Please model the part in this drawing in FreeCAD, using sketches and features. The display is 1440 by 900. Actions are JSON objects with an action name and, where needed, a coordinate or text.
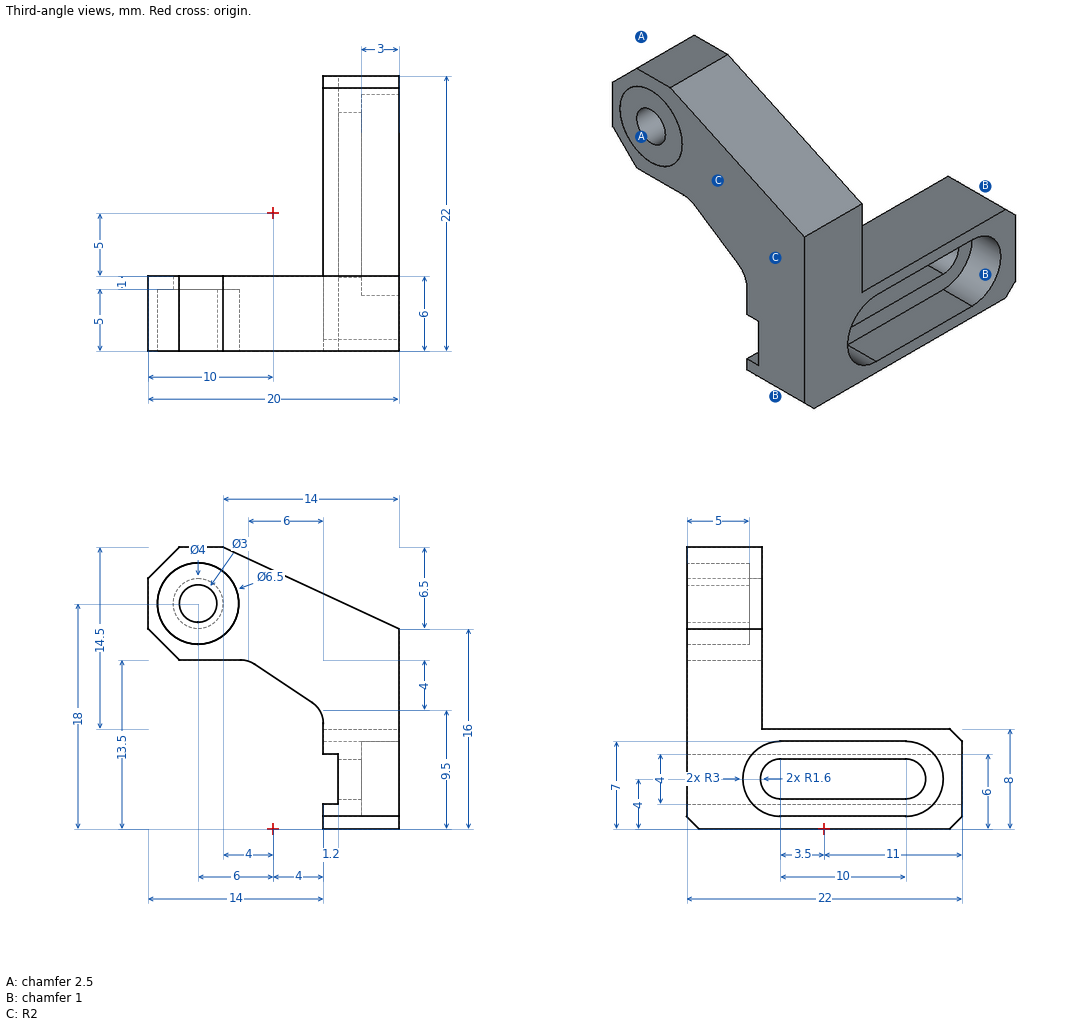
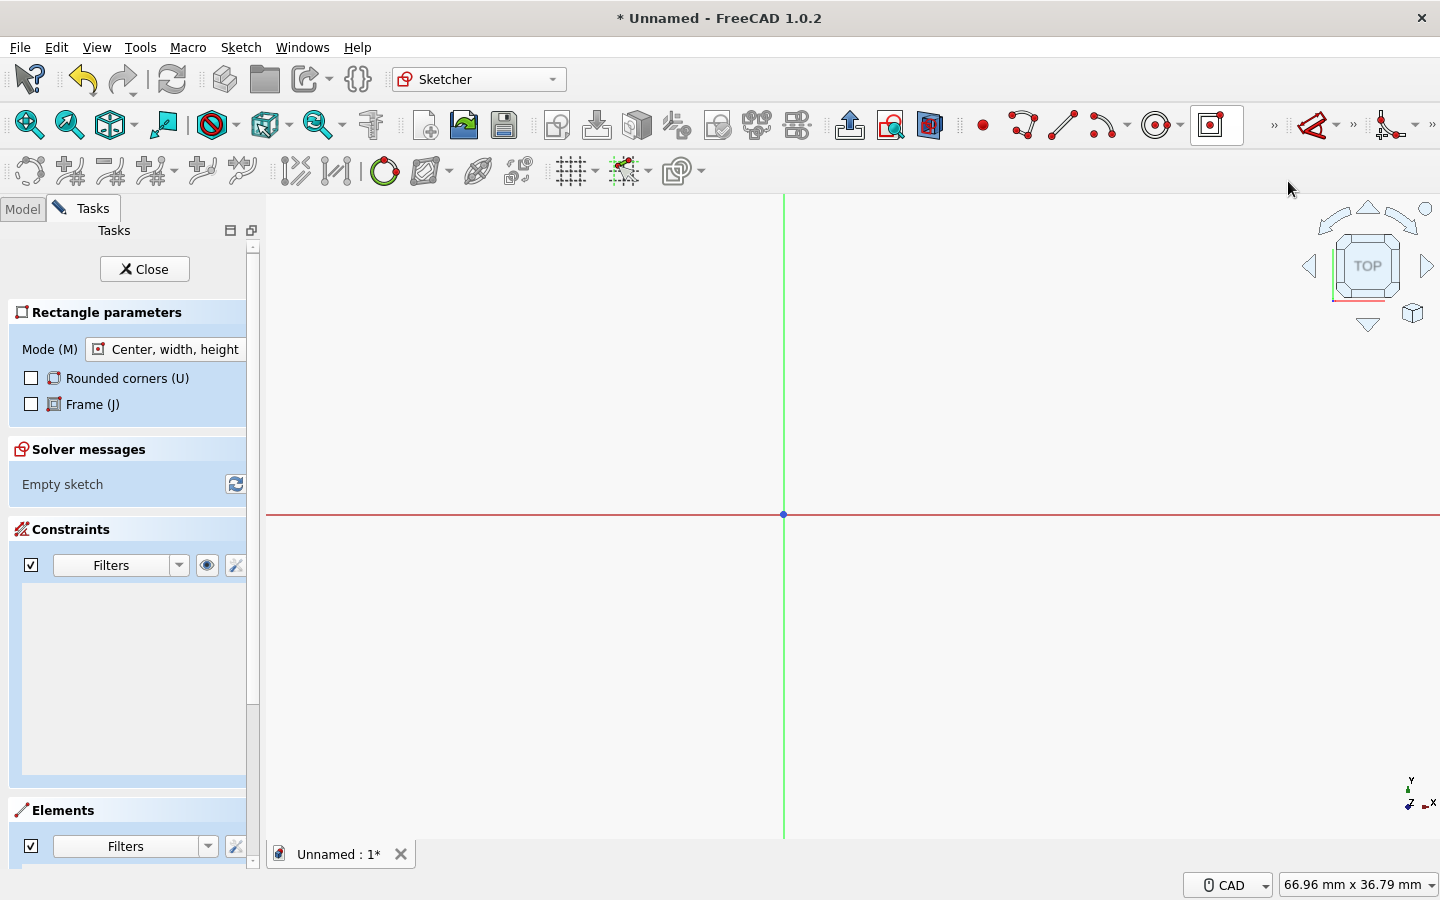
{"action": "left_click", "coordinate": [784, 515]}
{"action": "mouse_move", "coordinate": [959, 322]}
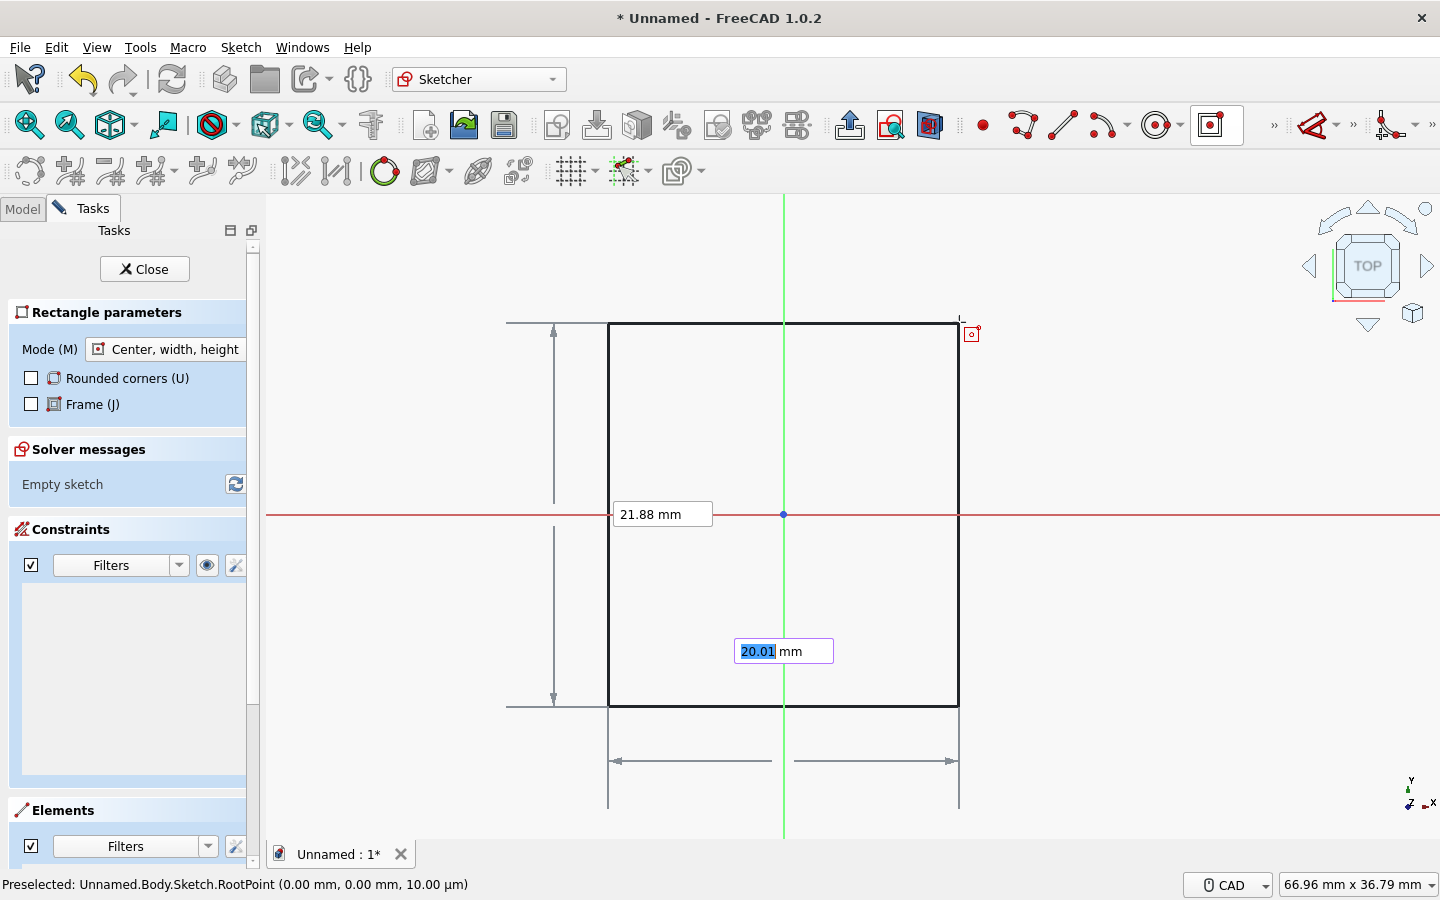
{"action": "type", "text": "20"}
{"action": "key", "text": "Tab"}
{"action": "type", "text": "22"}
{"action": "key", "text": "Return"}
{"action": "key", "text": "Escape"}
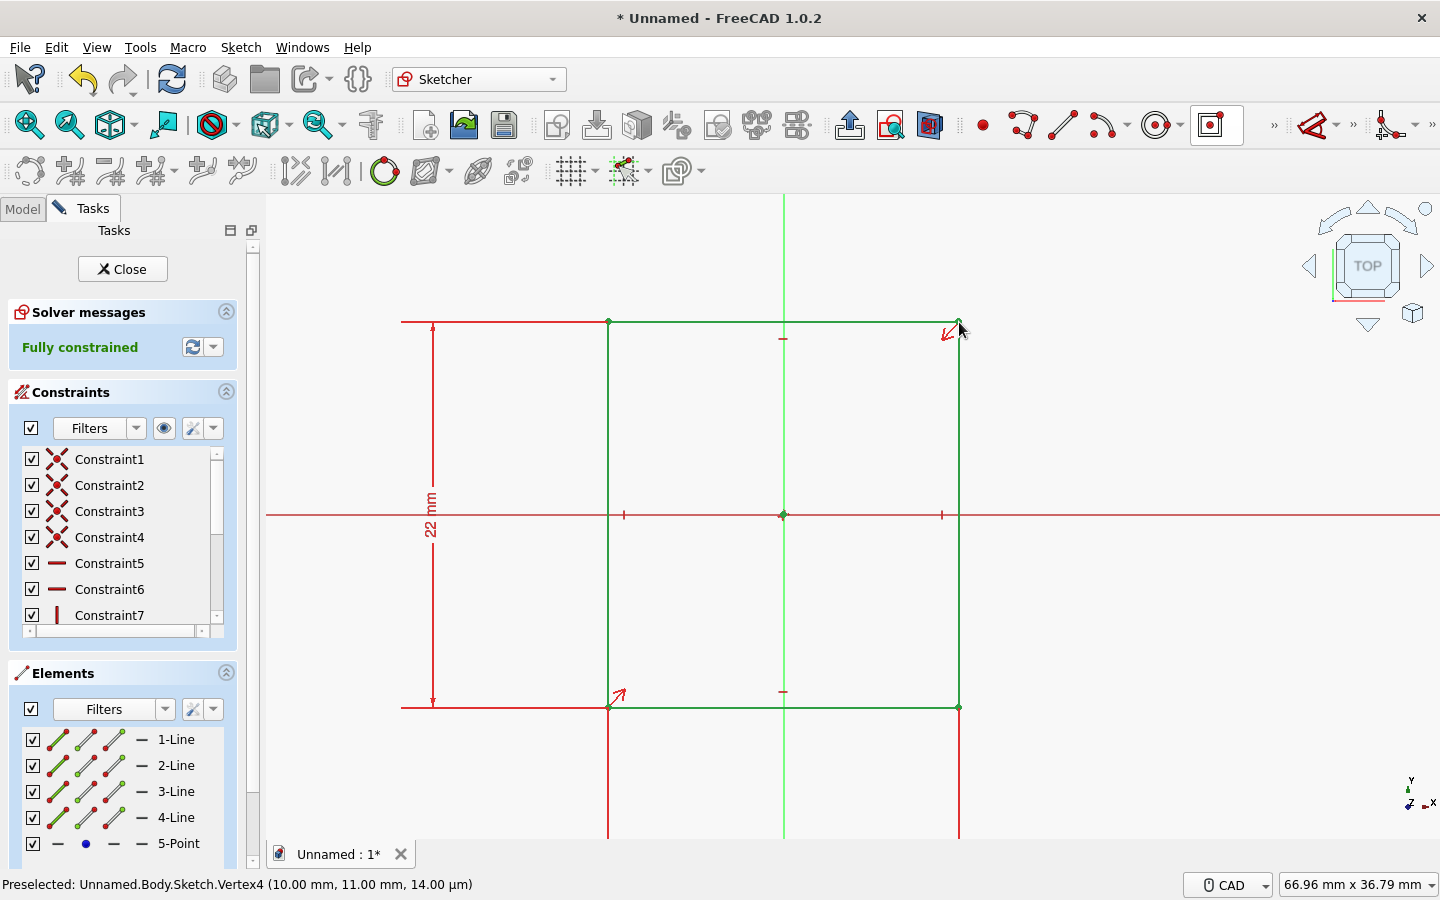
{"action": "left_click", "coordinate": [123, 269]}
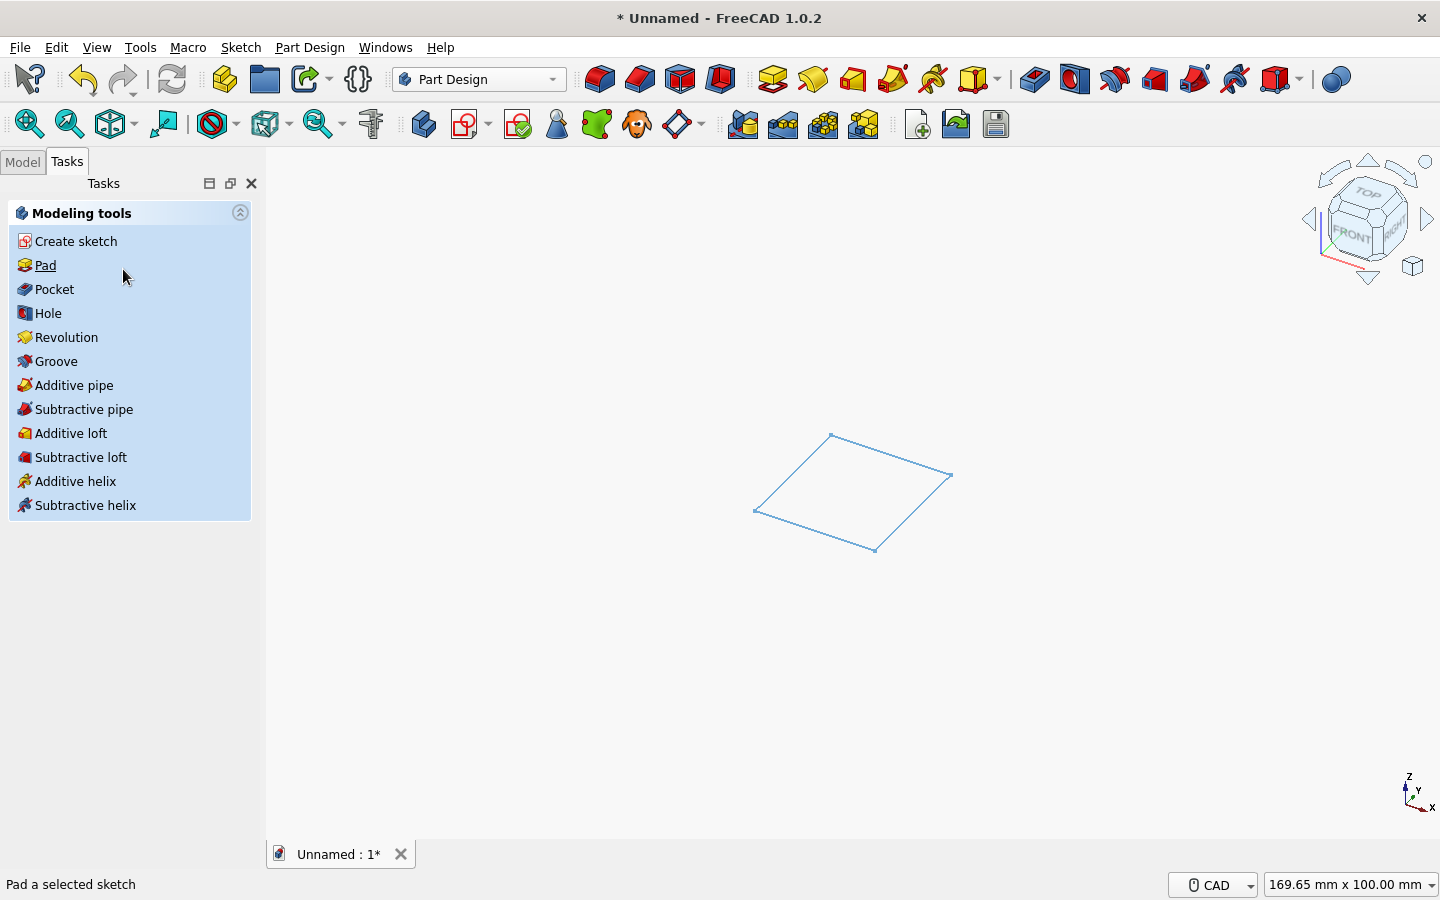
{"action": "left_click", "coordinate": [774, 80]}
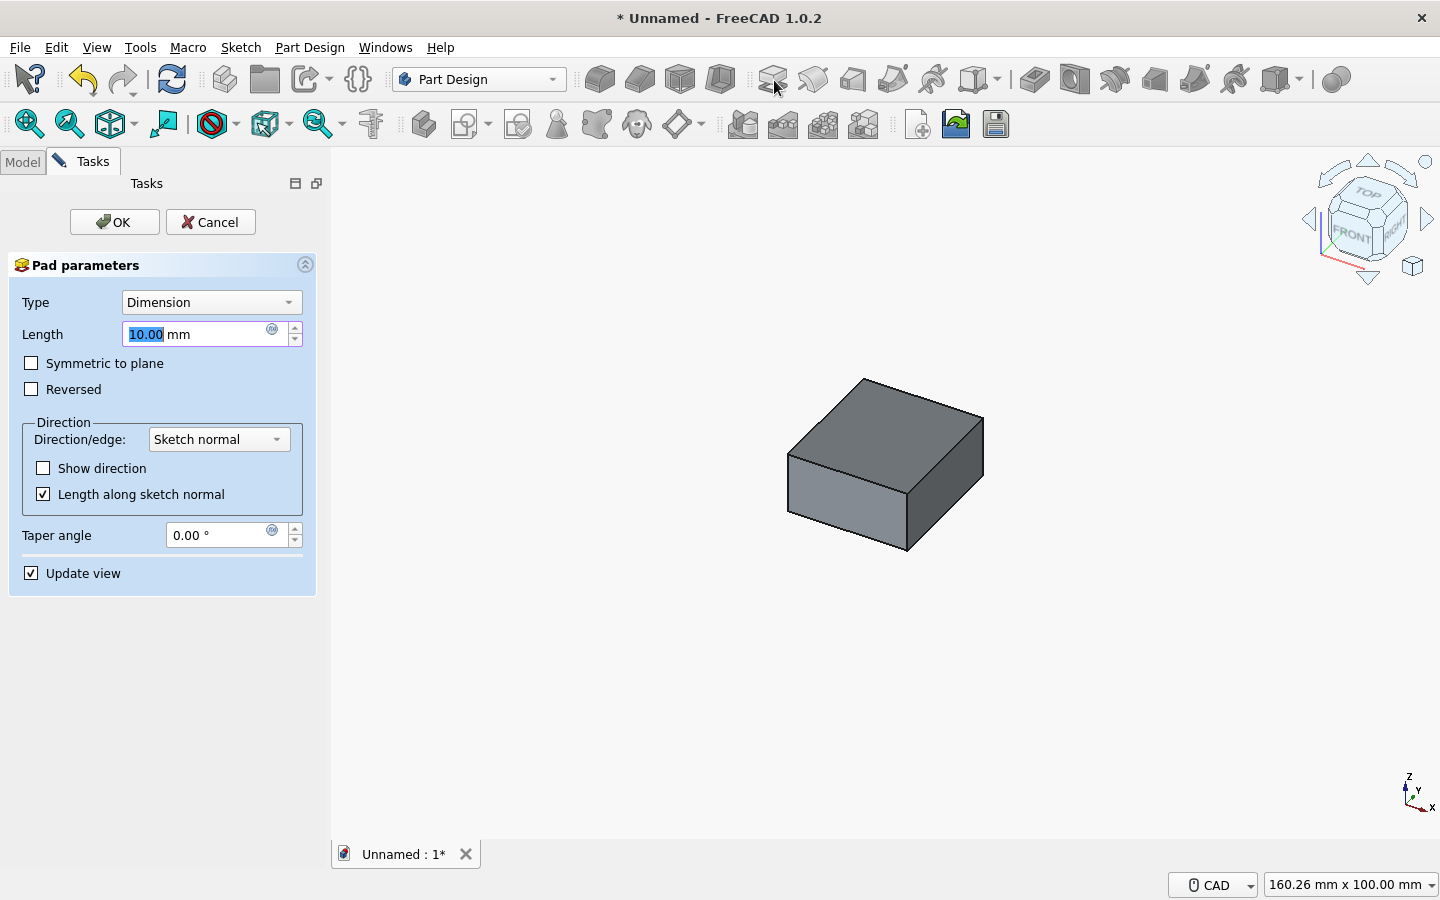
{"action": "type", "text": "8"}
{"action": "key", "text": "Tab"}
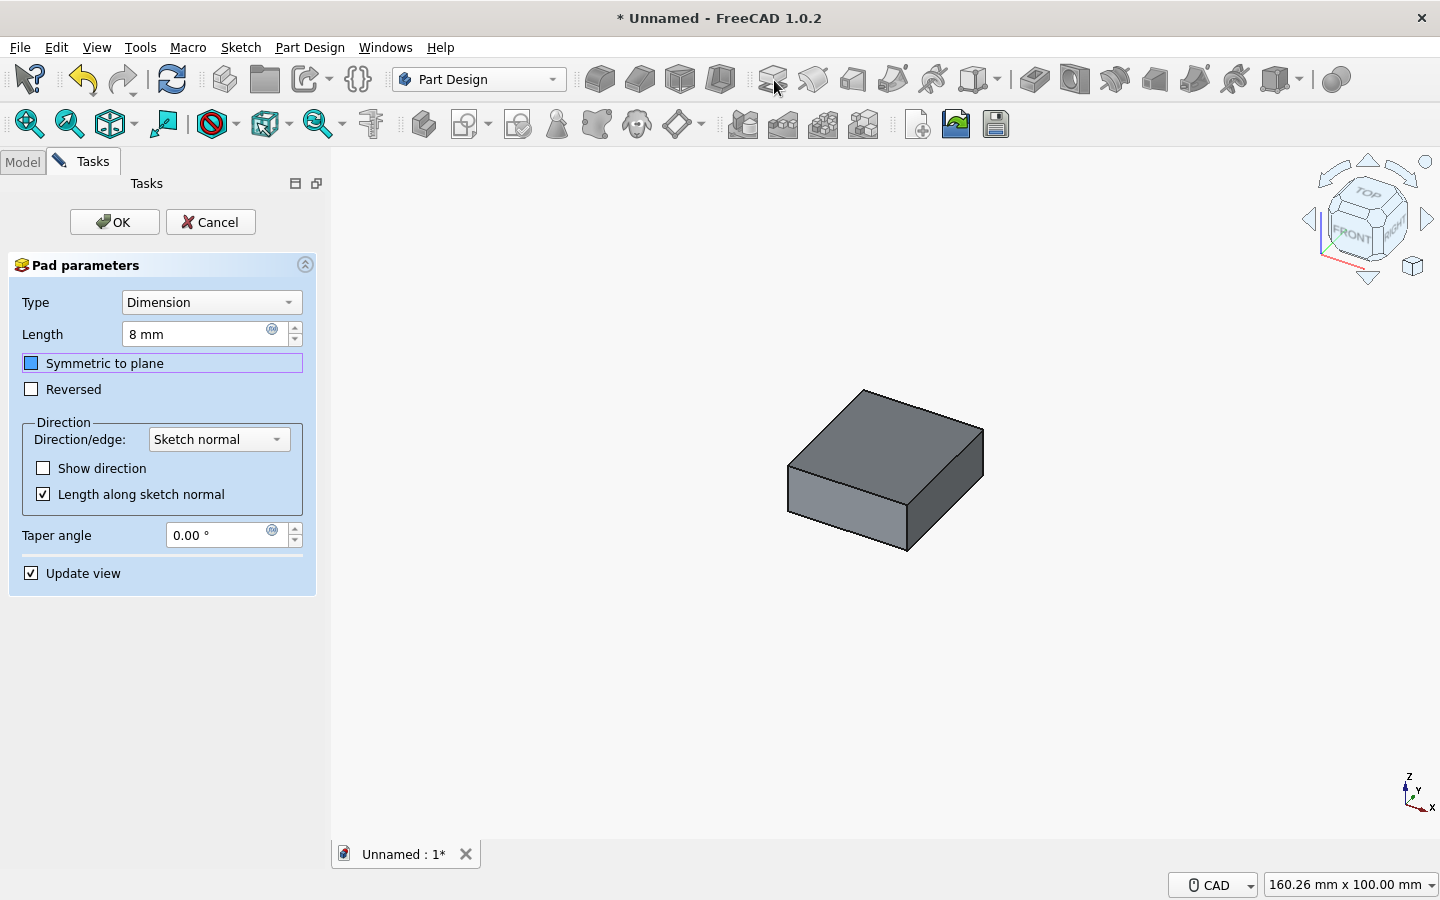
{"action": "left_click", "coordinate": [115, 222]}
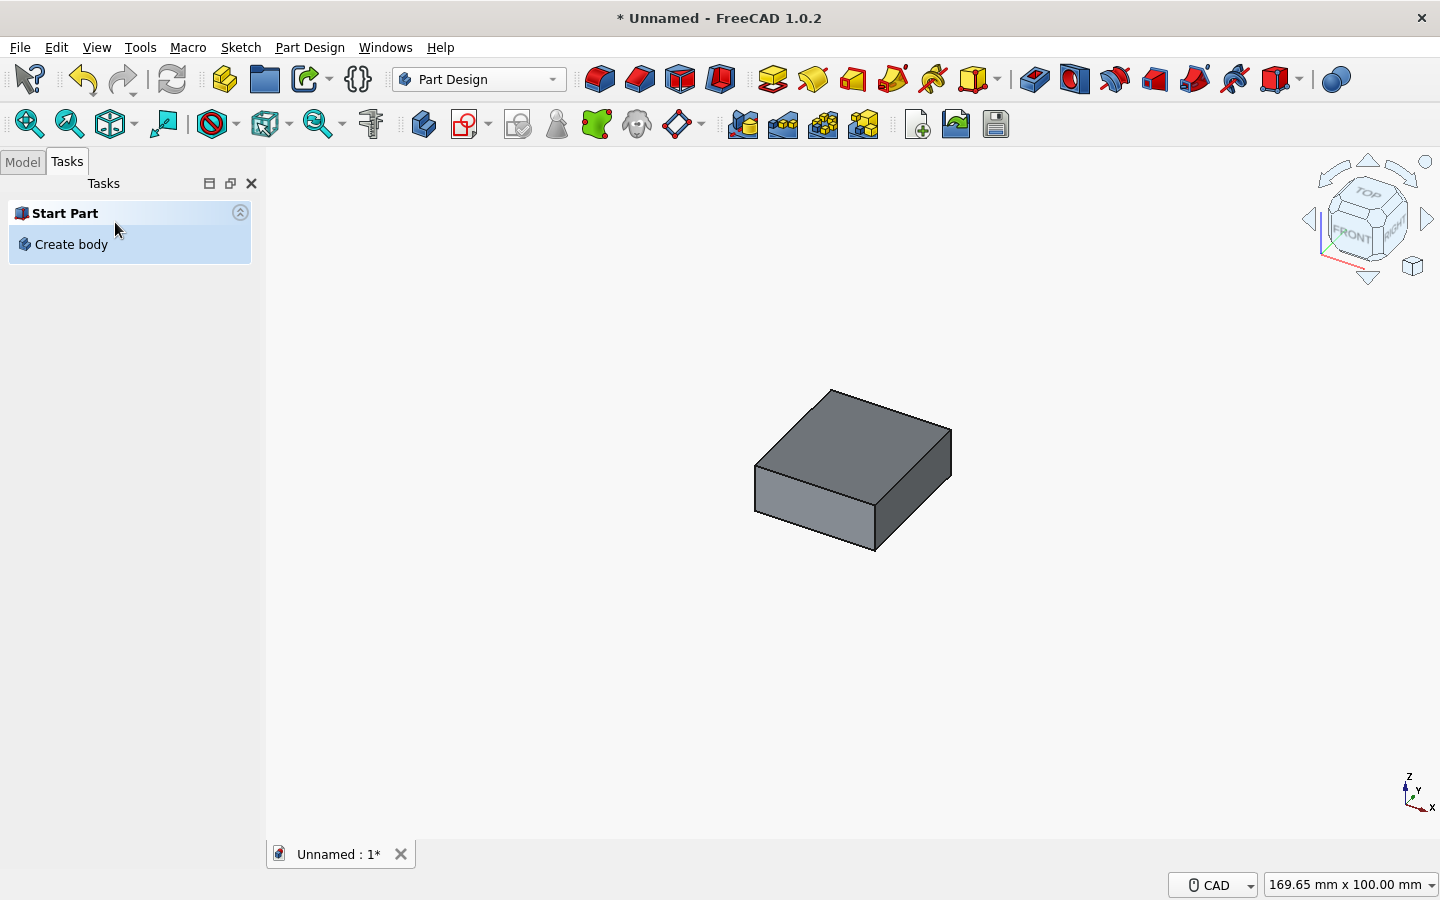
{"action": "left_click", "coordinate": [30, 124]}